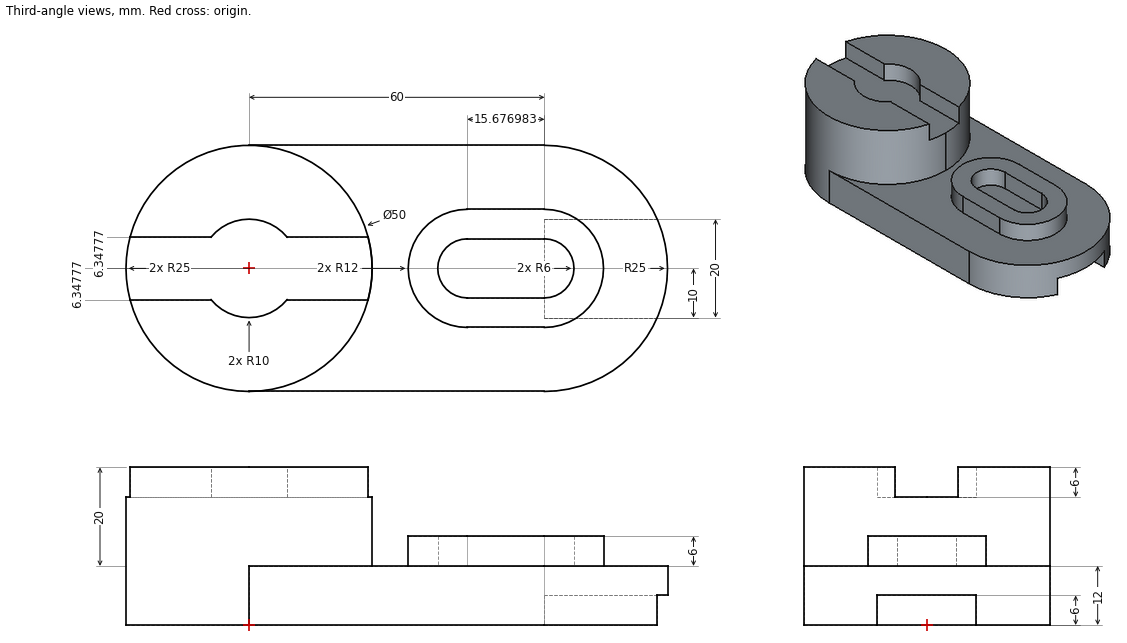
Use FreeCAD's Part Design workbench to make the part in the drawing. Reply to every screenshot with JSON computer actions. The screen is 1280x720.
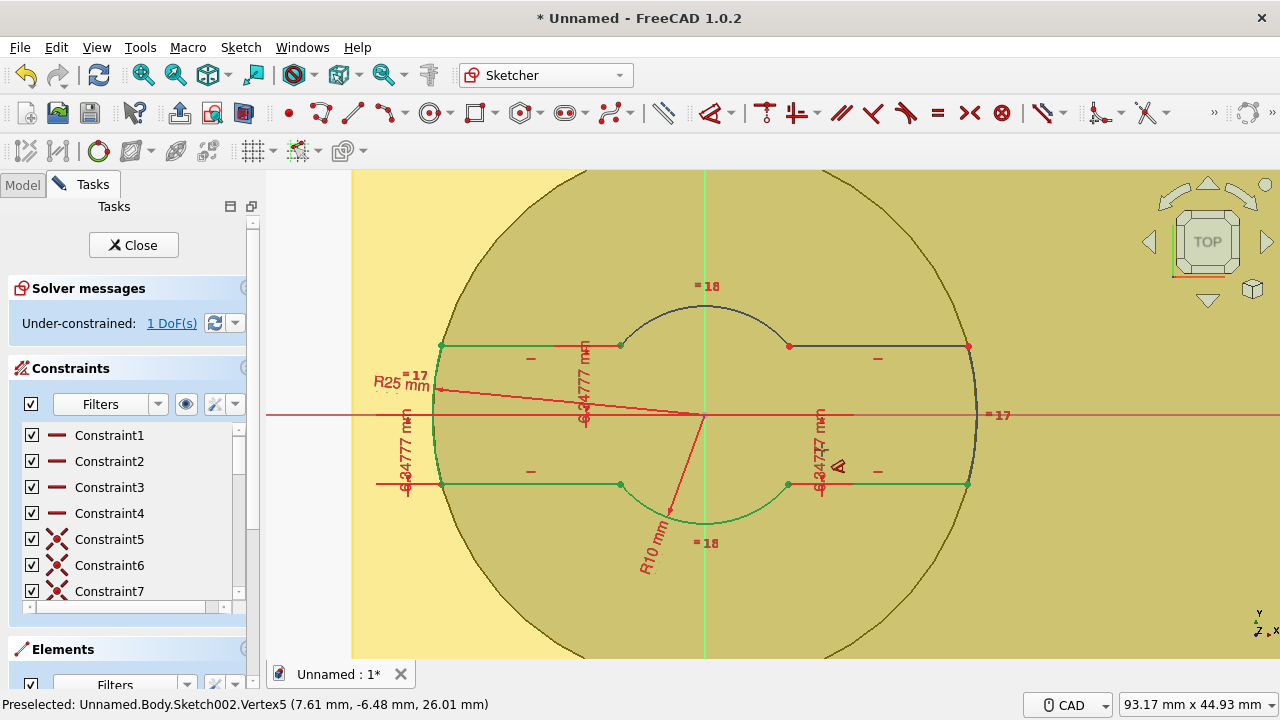
{"action": "left_click", "coordinate": [968, 346]}
{"action": "left_click", "coordinate": [1002, 381]}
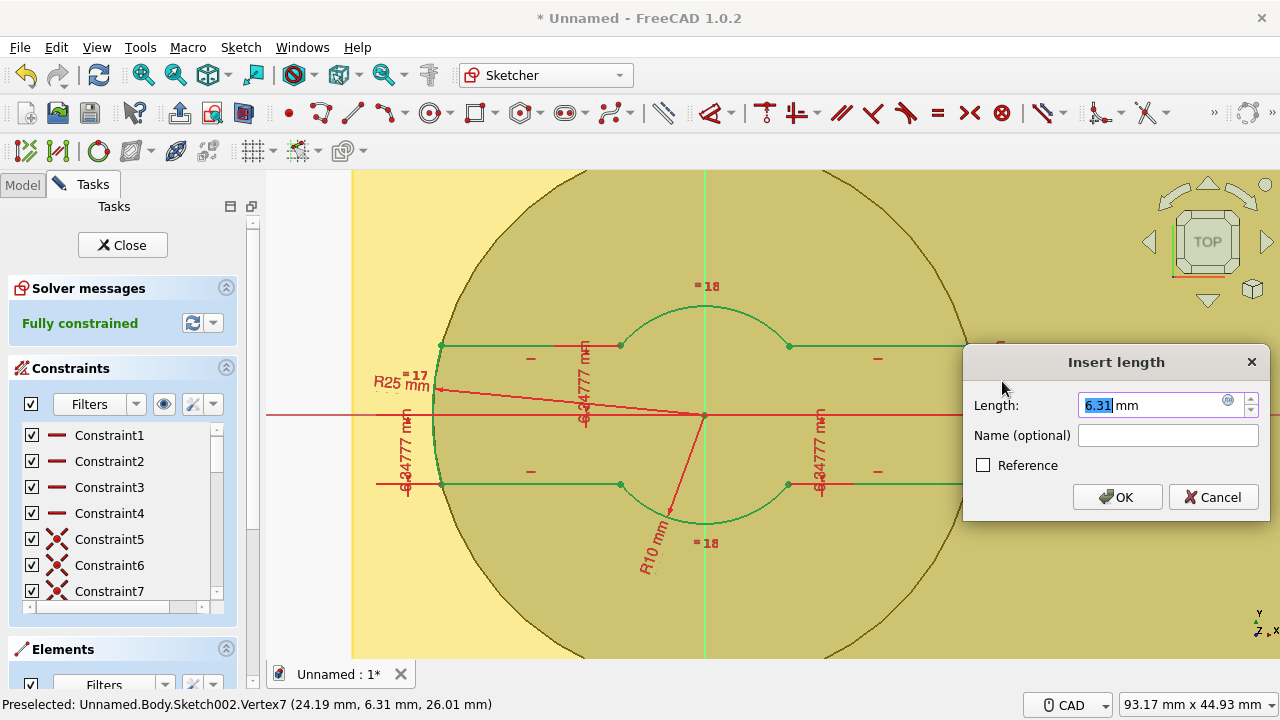
{"action": "type", "text": "6.34777"}
{"action": "key", "text": "Return"}
{"action": "key", "text": "Escape"}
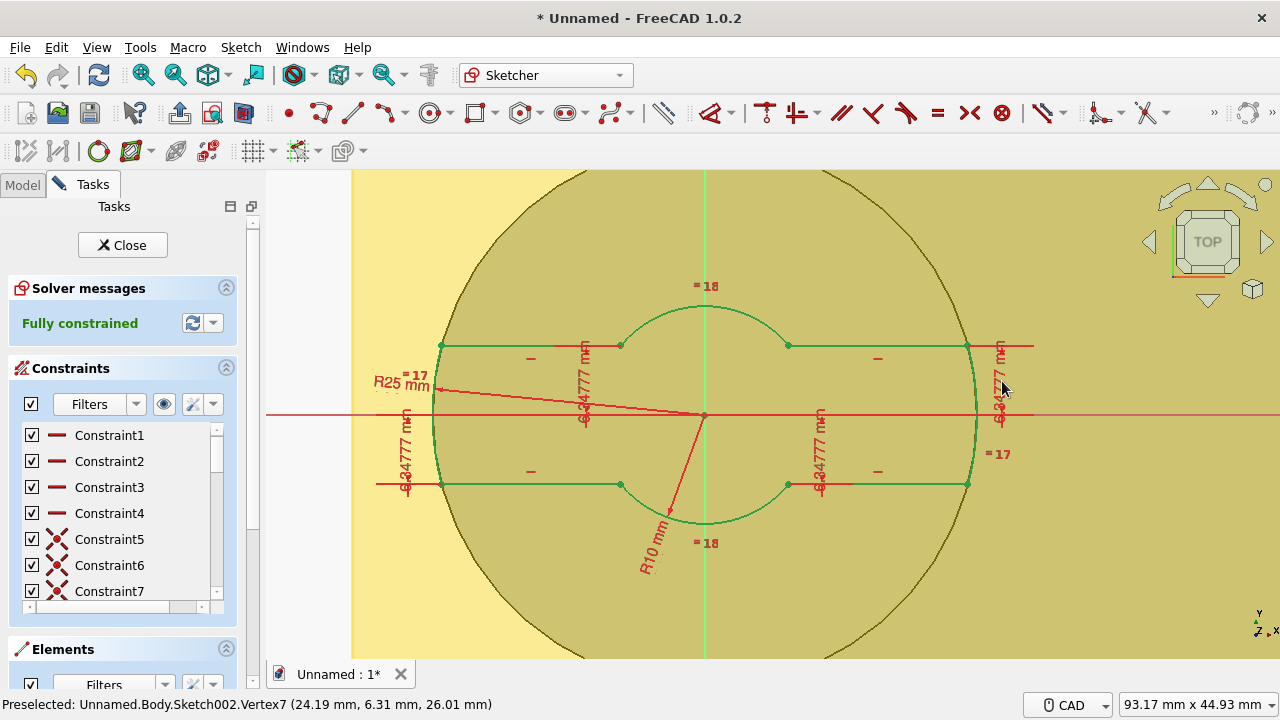
{"action": "left_click", "coordinate": [123, 245]}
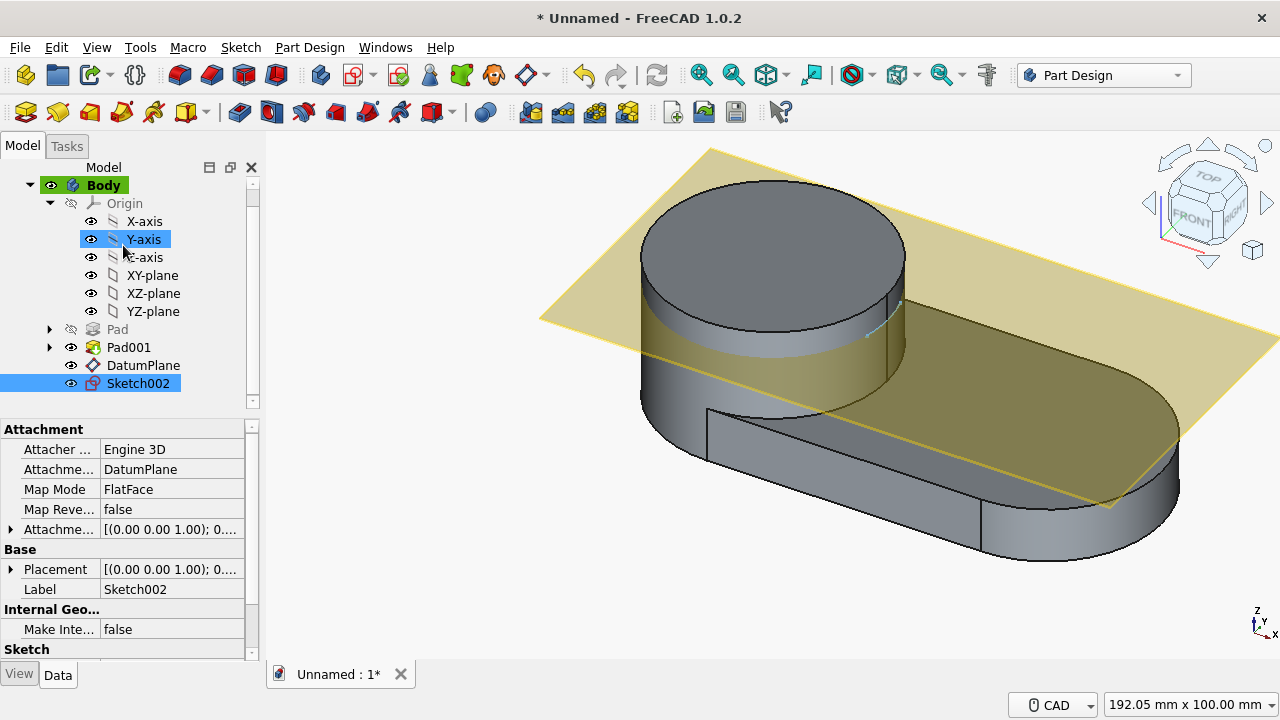
{"action": "left_click", "coordinate": [240, 112]}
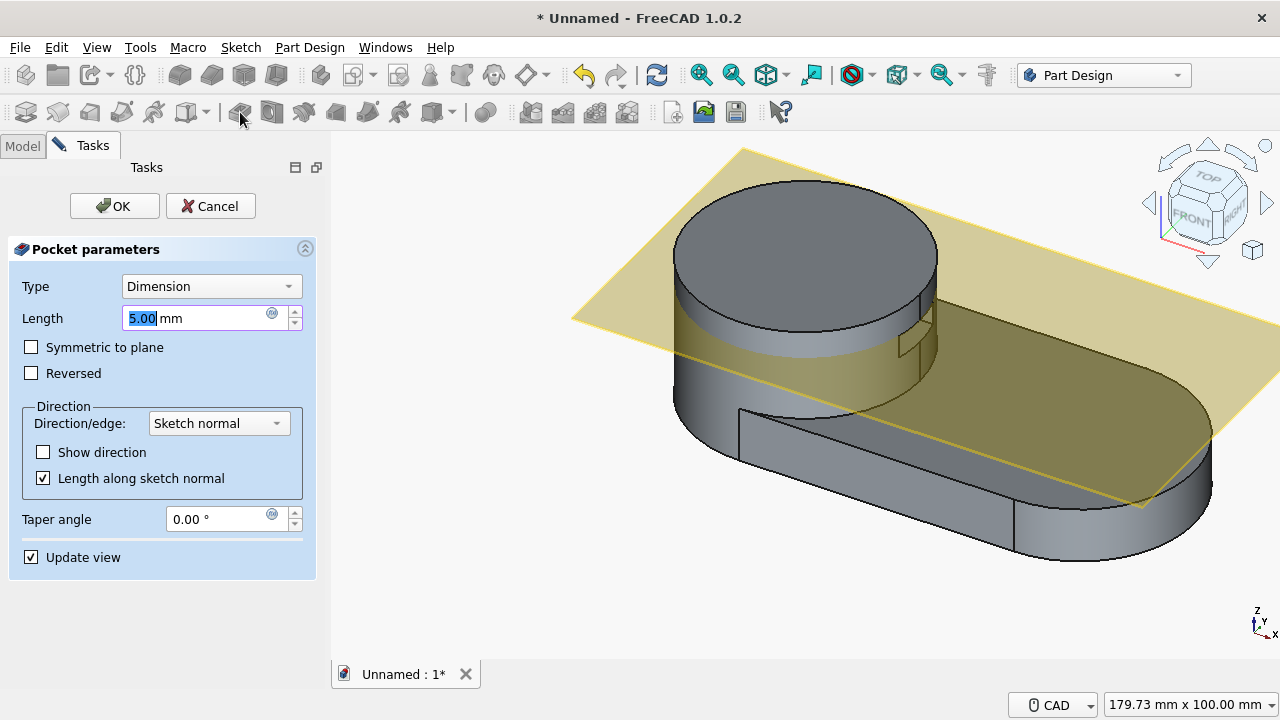
{"action": "type", "text": "6"}
{"action": "key", "text": "Tab"}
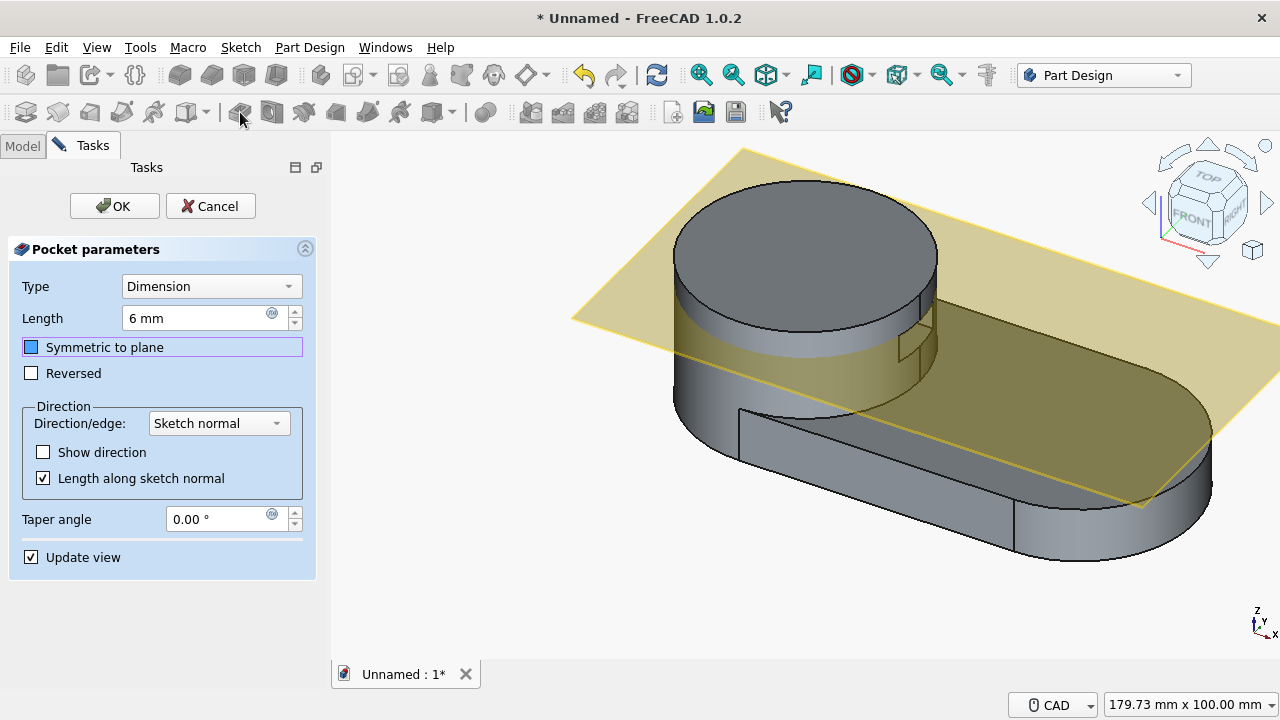
{"action": "left_click", "coordinate": [30, 373]}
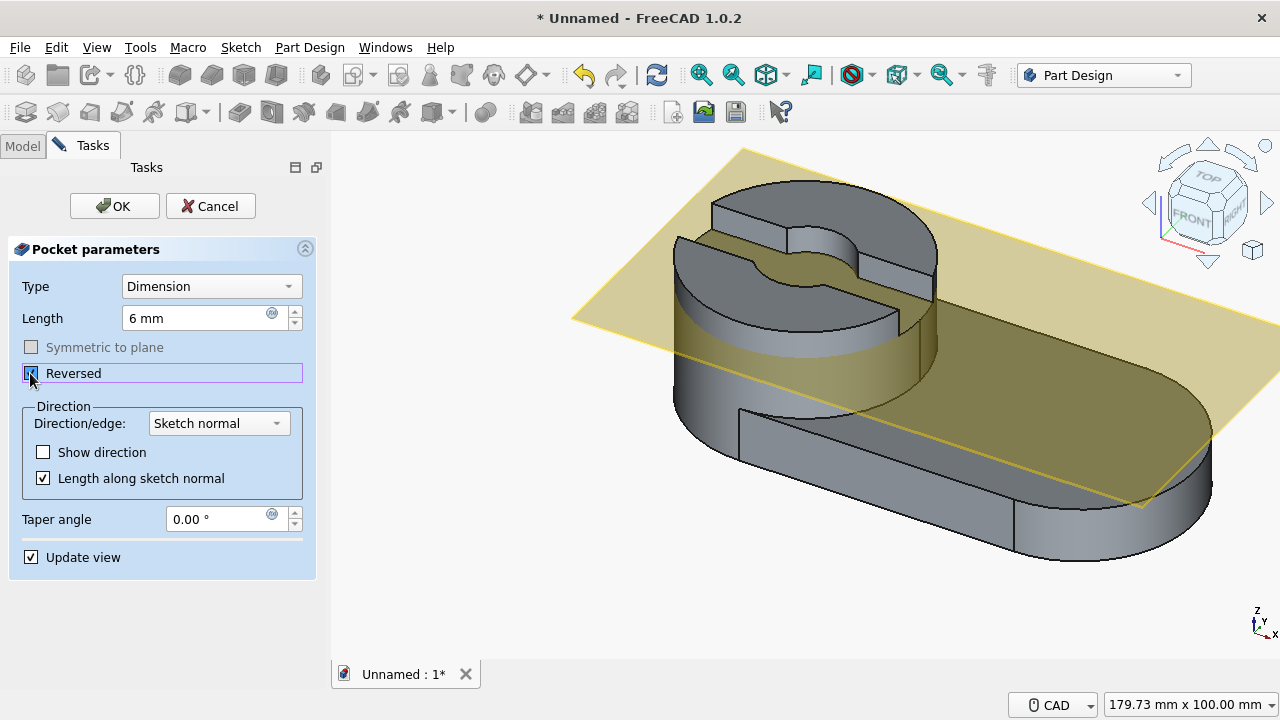
{"action": "left_click", "coordinate": [115, 206]}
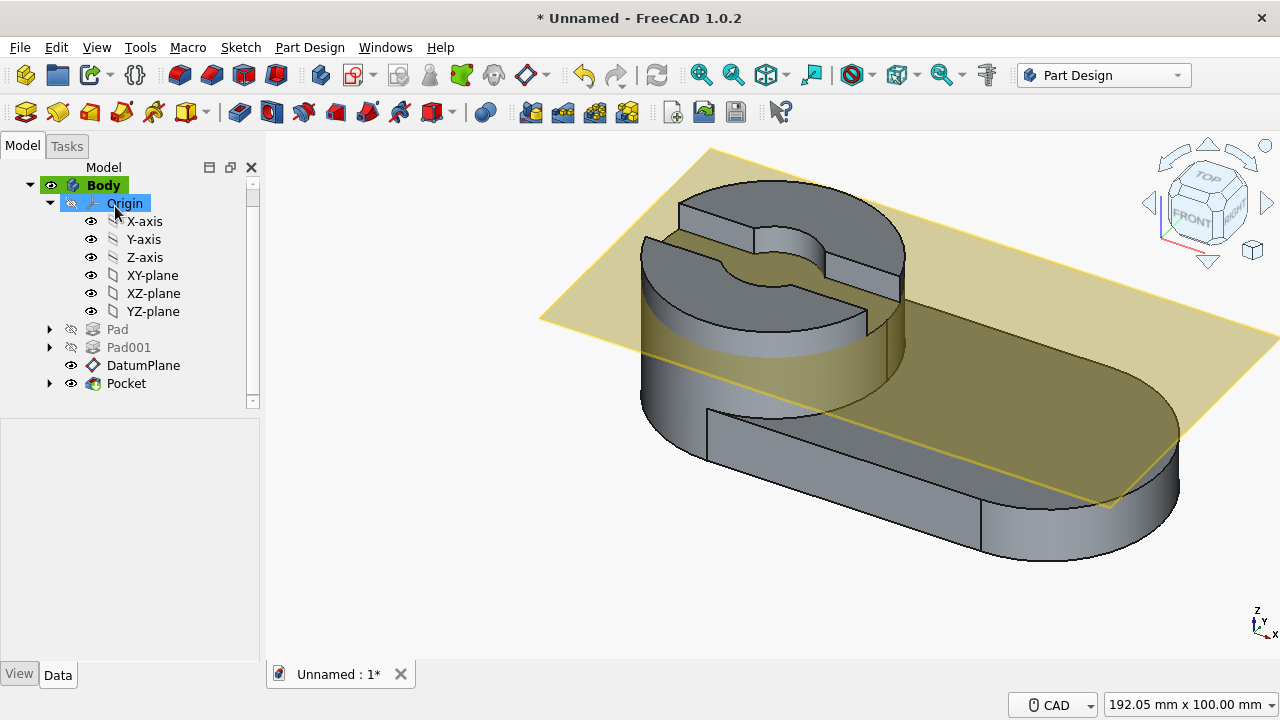
{"action": "left_click", "coordinate": [116, 365]}
{"action": "key", "text": "space"}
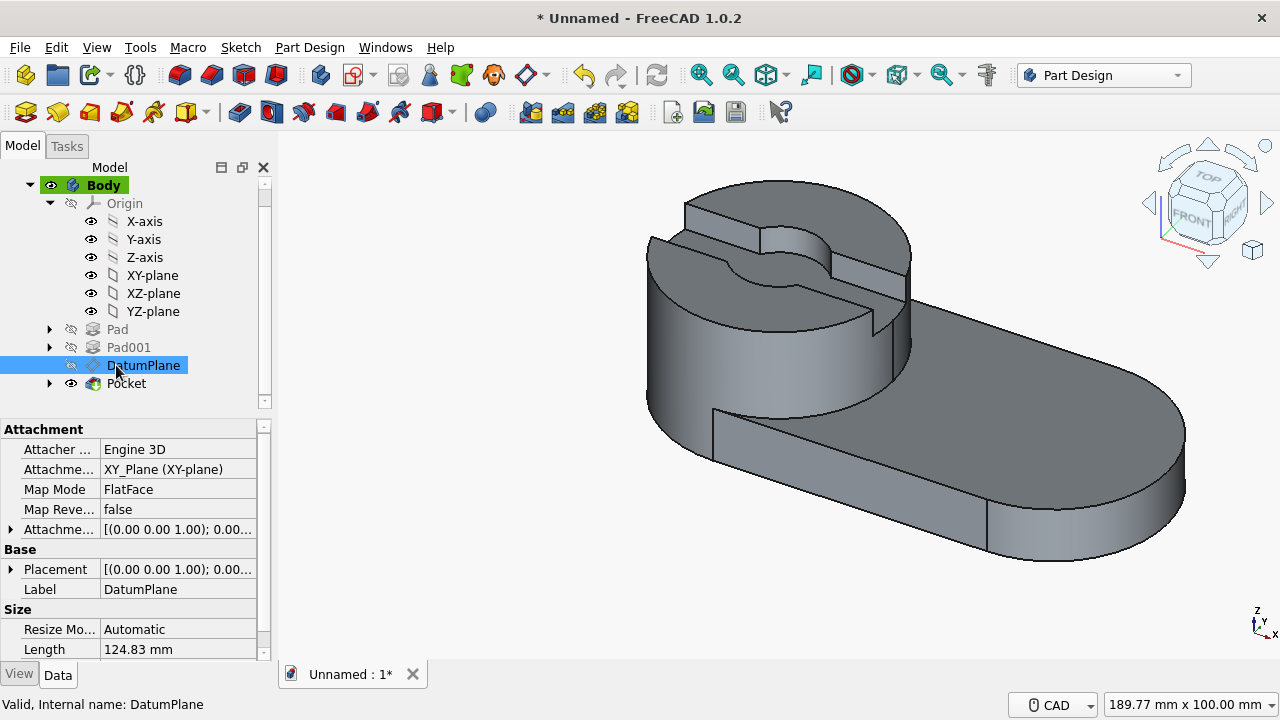
{"action": "left_click", "coordinate": [1029, 425]}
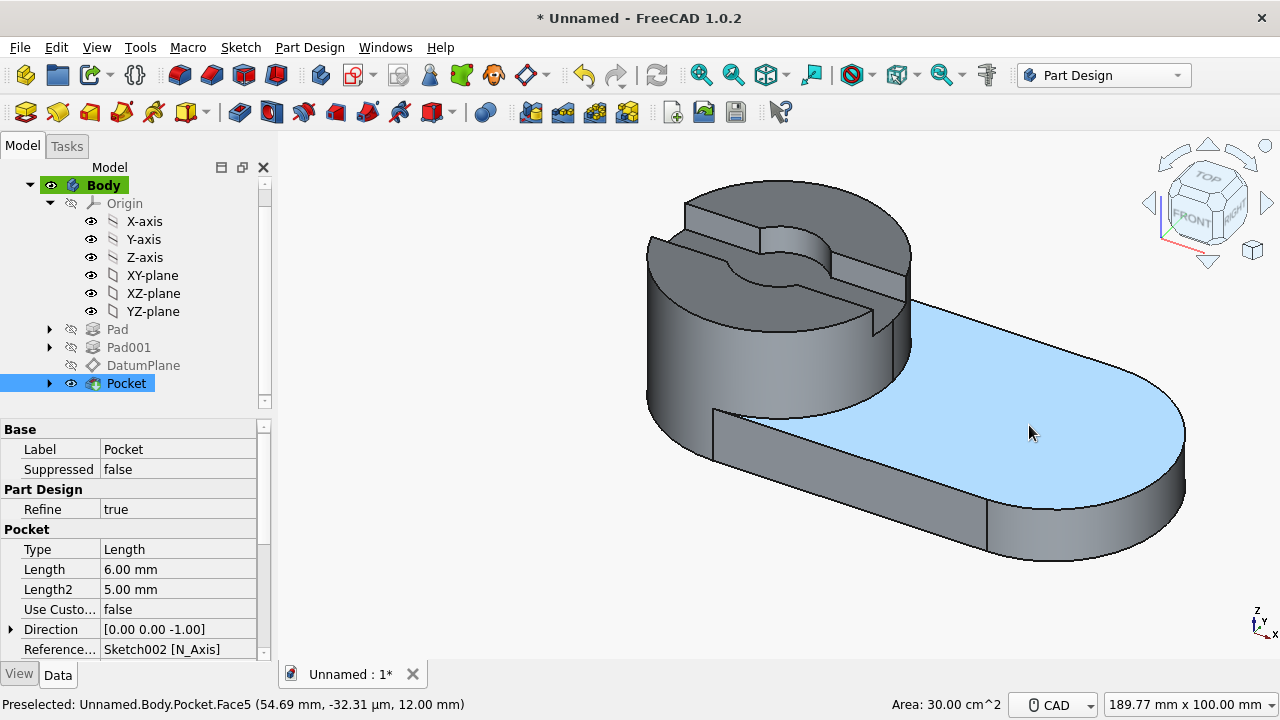
{"action": "left_click", "coordinate": [354, 76]}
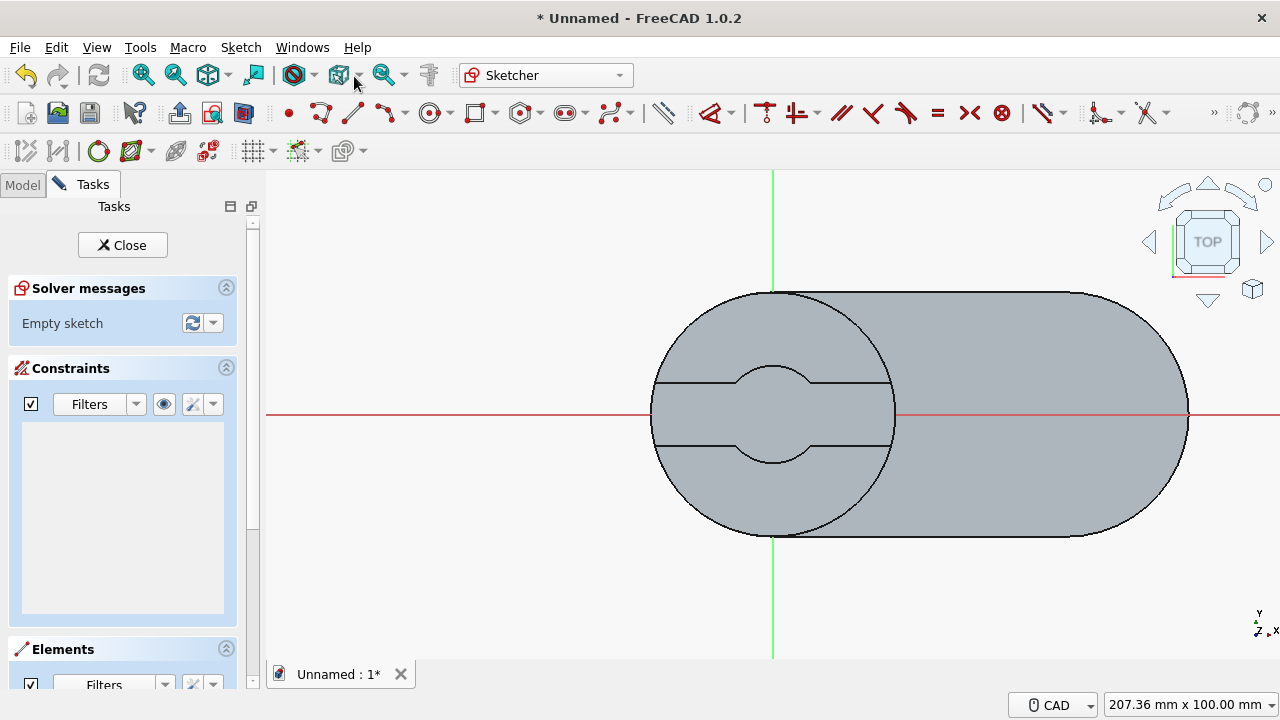
{"action": "left_click", "coordinate": [244, 114]}